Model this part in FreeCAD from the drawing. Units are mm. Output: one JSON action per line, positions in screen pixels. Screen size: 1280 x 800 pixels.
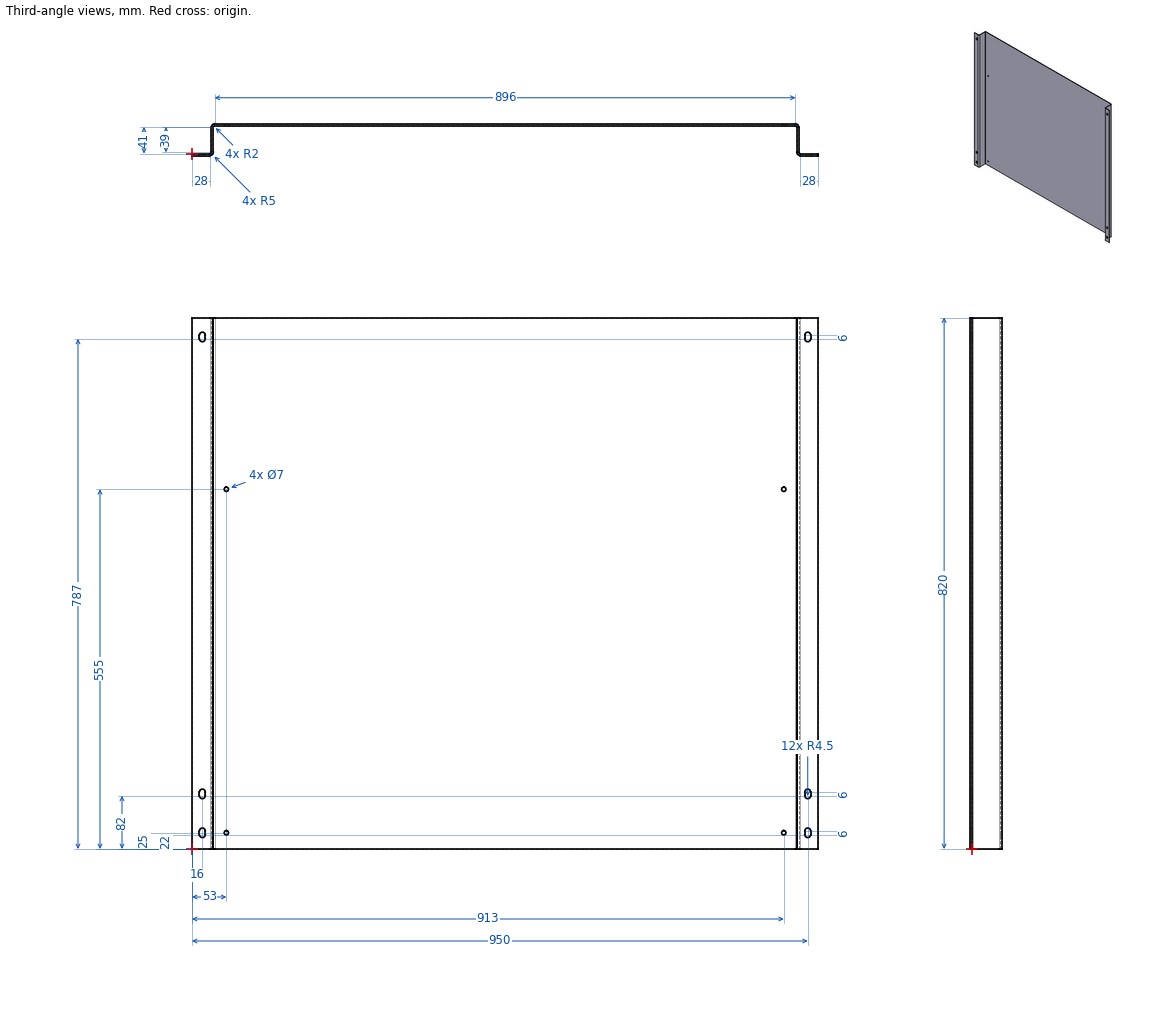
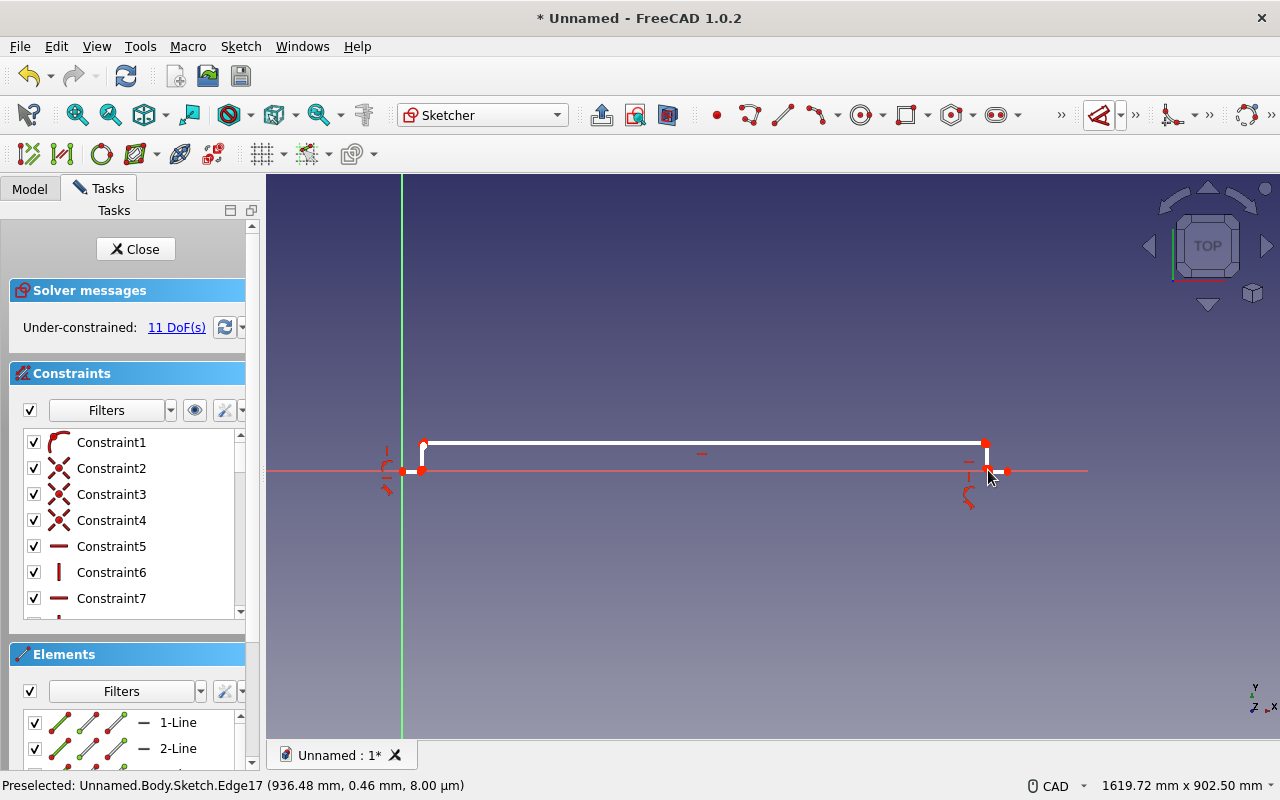
{"action": "scroll", "coordinate": [421, 470], "scroll_direction": "up", "scroll_amount": 14}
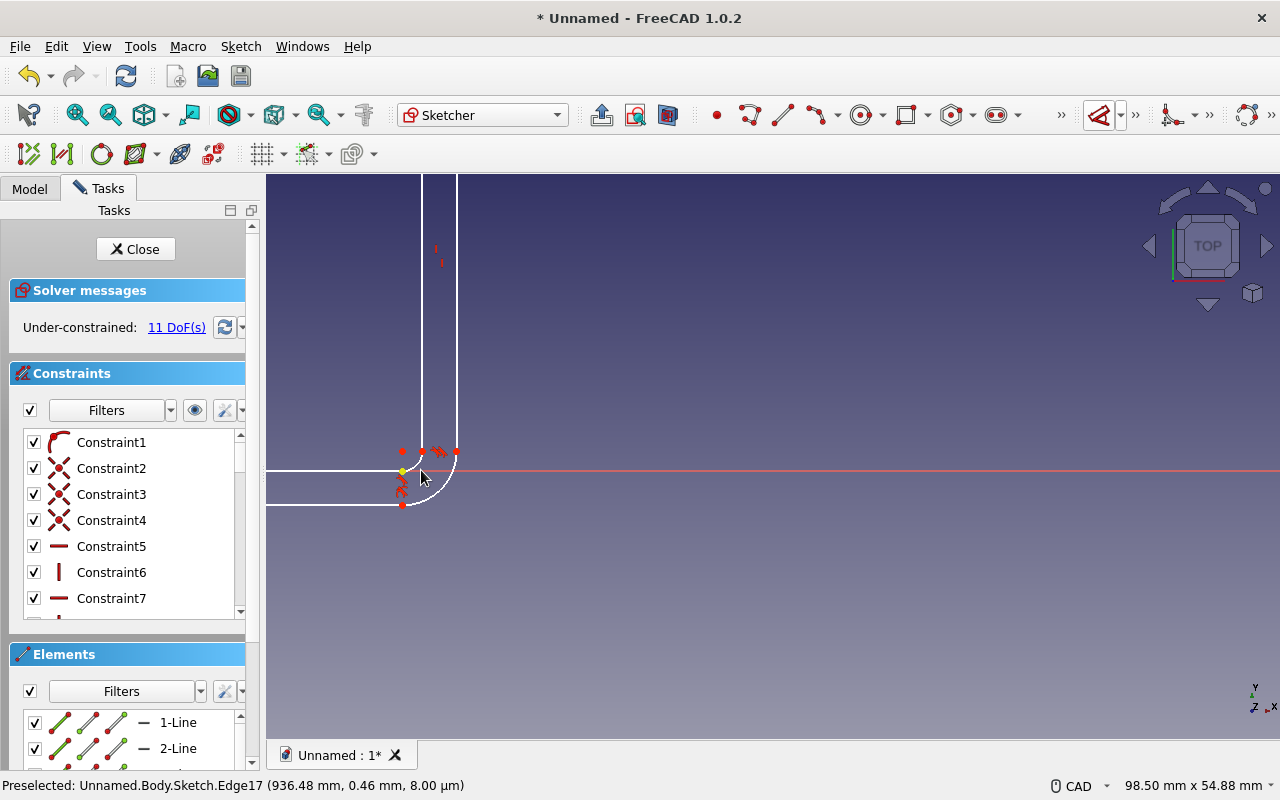
{"action": "left_click", "coordinate": [412, 469]}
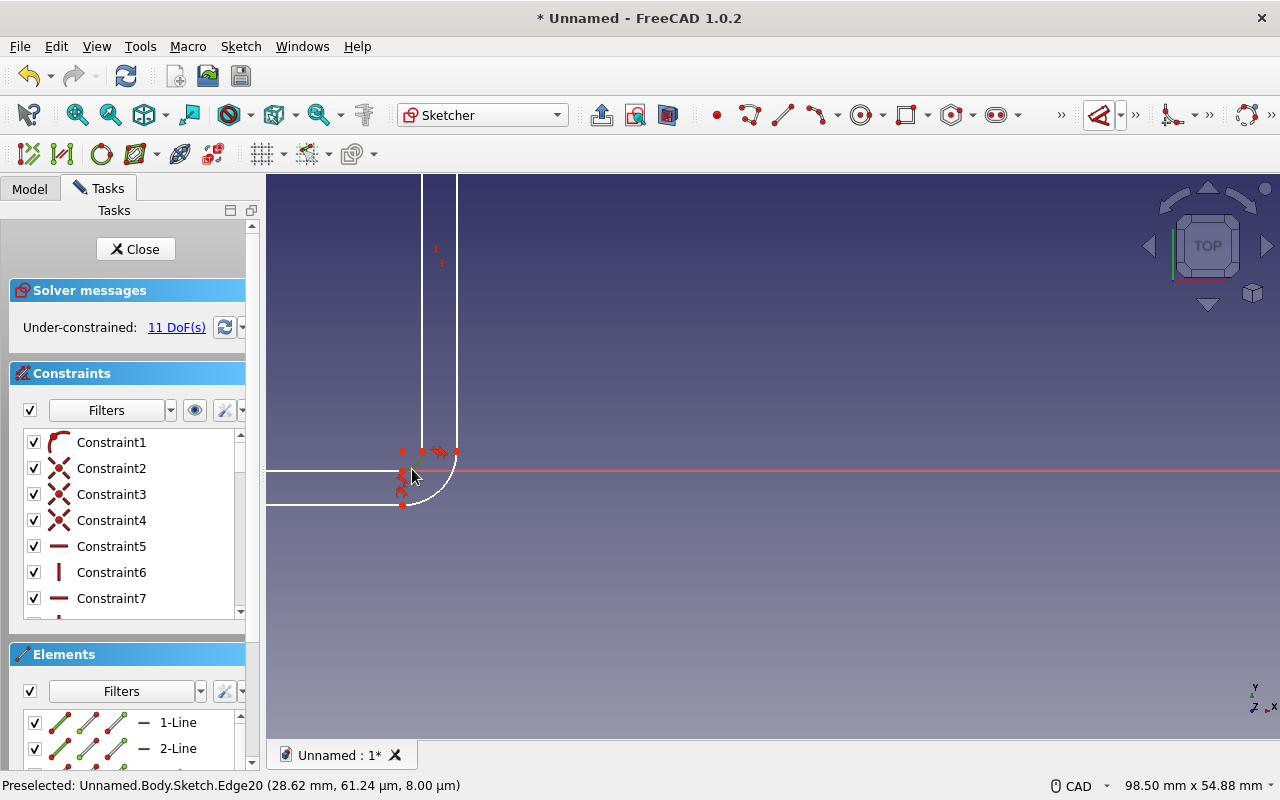
{"action": "key", "text": "e"}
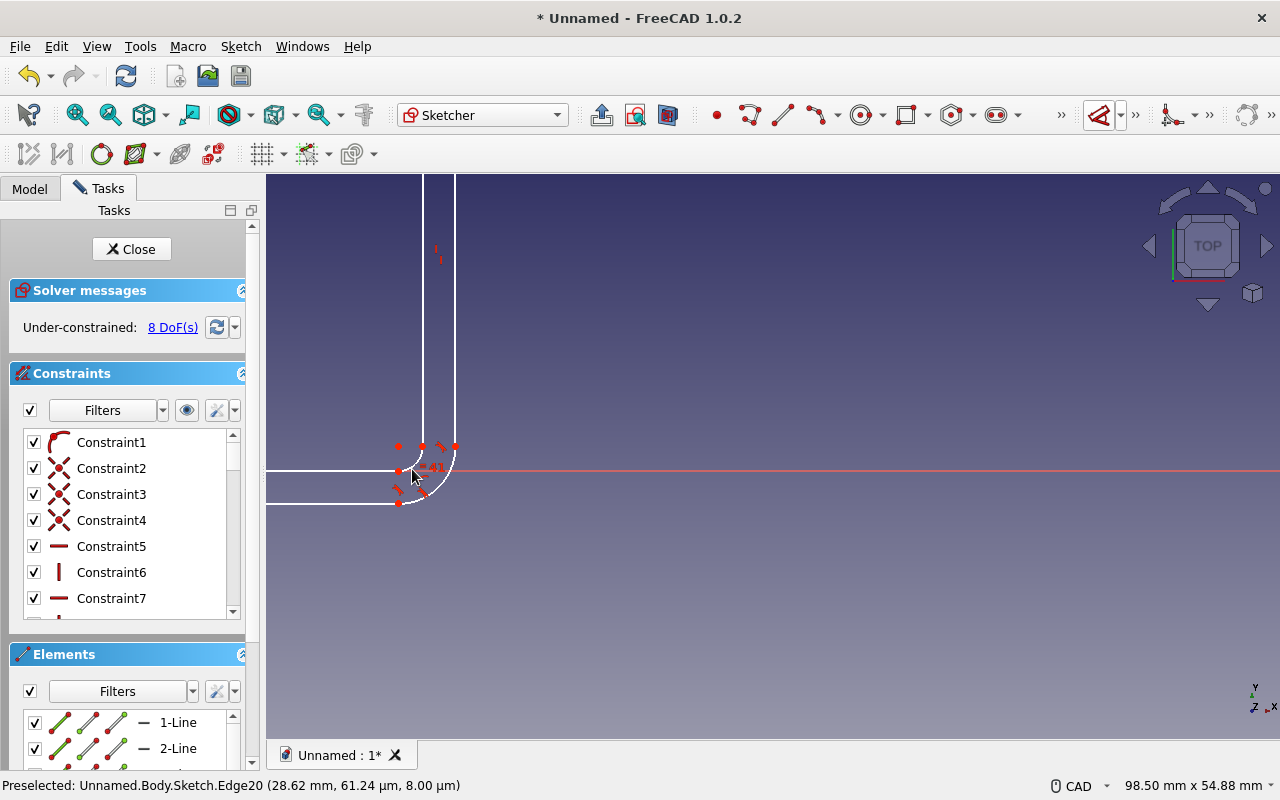
{"action": "key", "text": "d"}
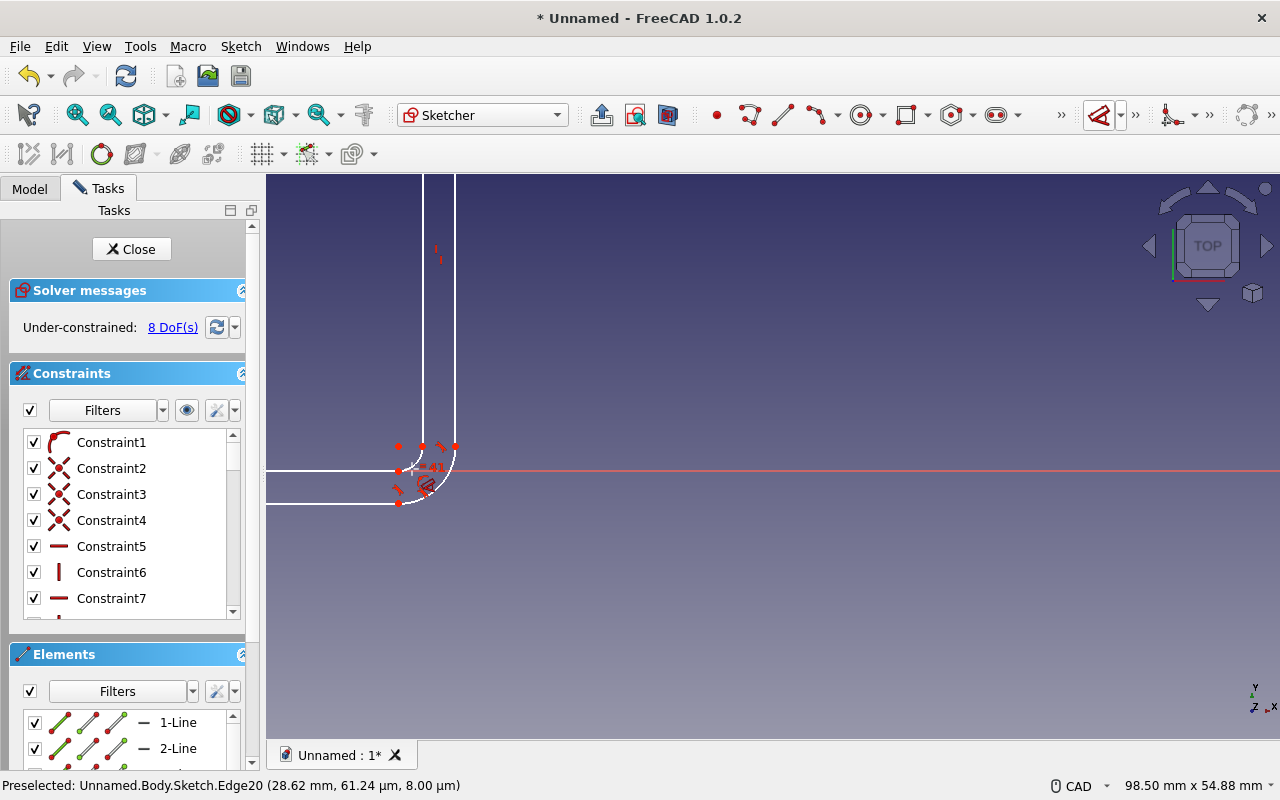
{"action": "left_click", "coordinate": [424, 498]}
{"action": "left_click", "coordinate": [438, 527]}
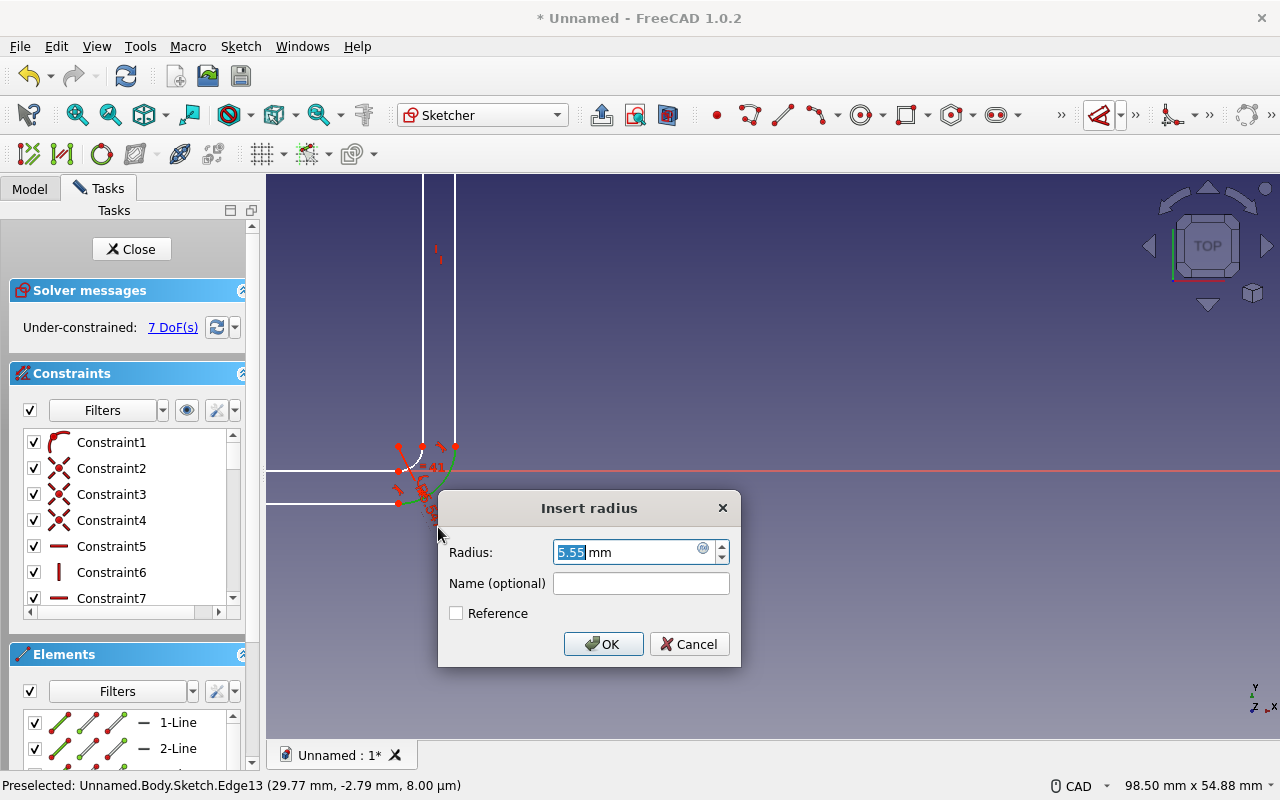
{"action": "type", "text": "5"}
{"action": "key", "text": "Return"}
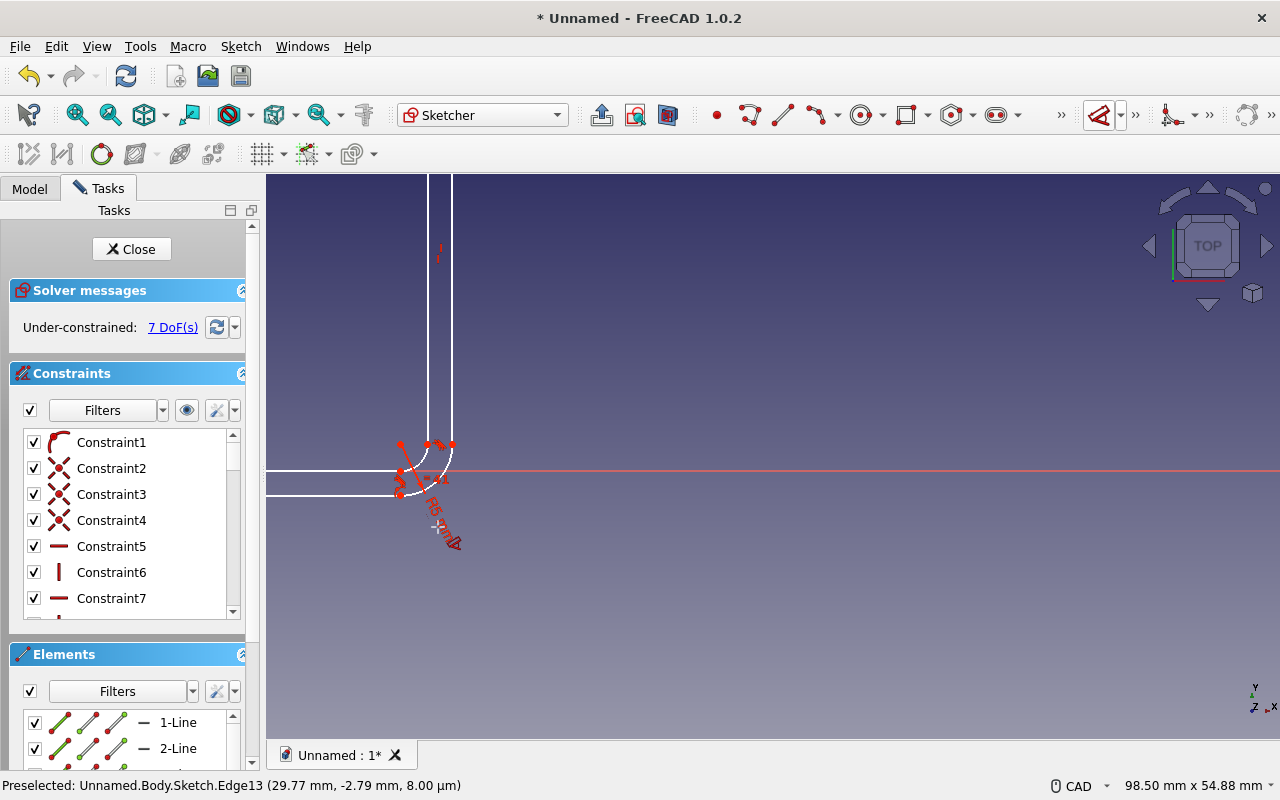
{"action": "scroll", "coordinate": [421, 470], "scroll_direction": "down", "scroll_amount": 14}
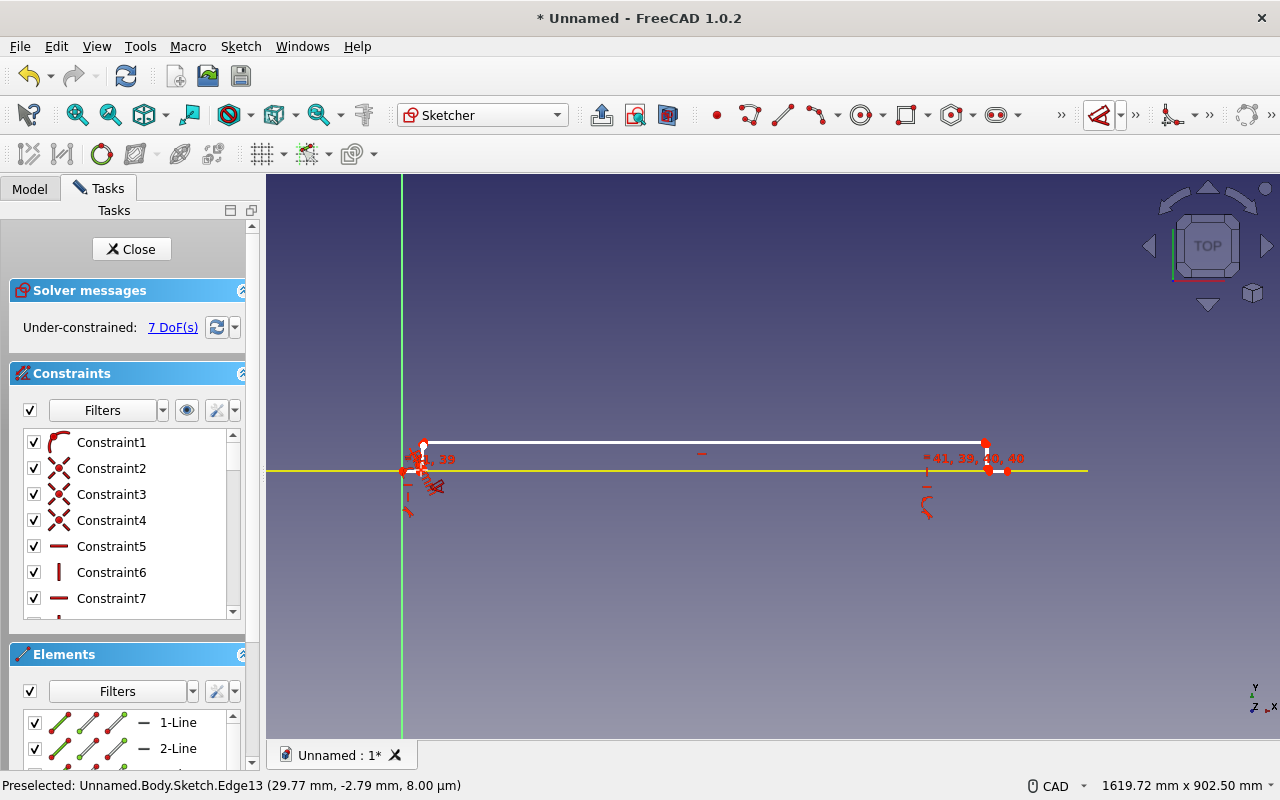
{"action": "scroll", "coordinate": [424, 444], "scroll_direction": "up", "scroll_amount": 18}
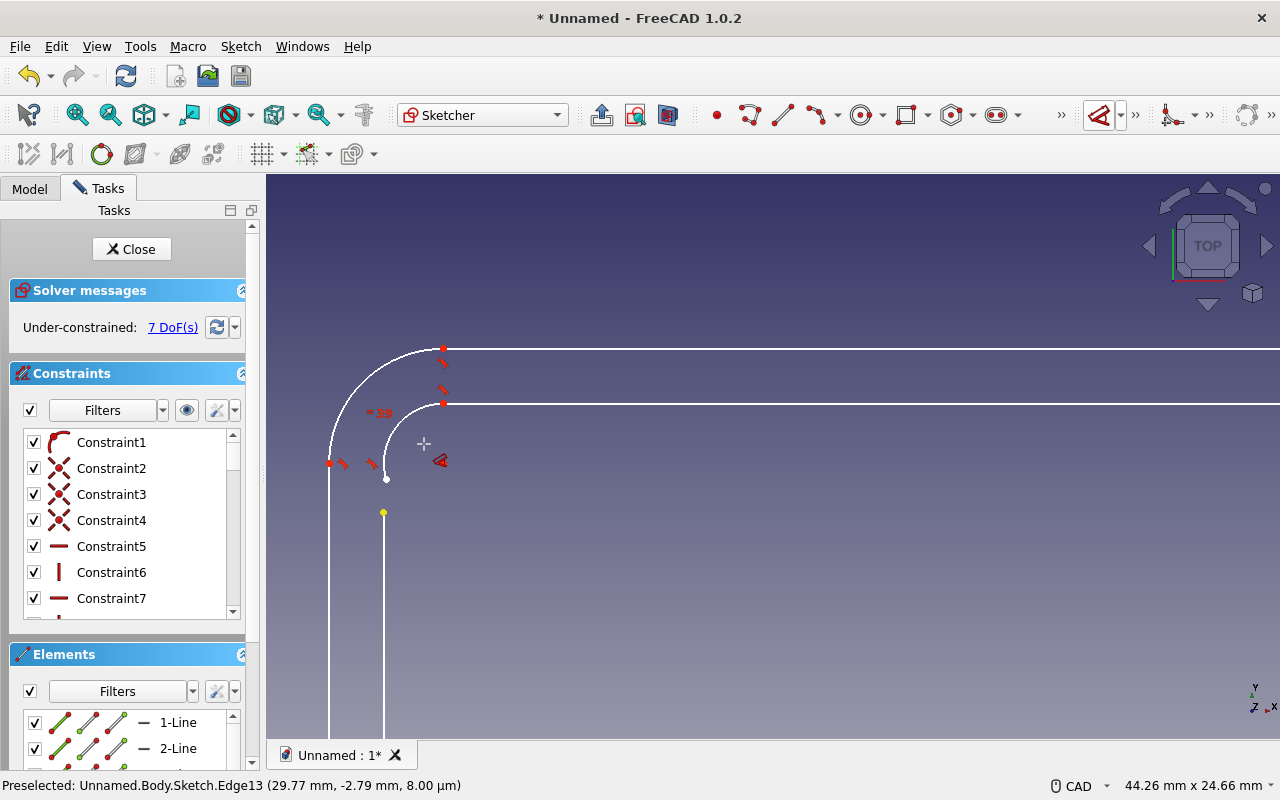
{"action": "left_click", "coordinate": [412, 413]}
{"action": "left_click", "coordinate": [395, 386]}